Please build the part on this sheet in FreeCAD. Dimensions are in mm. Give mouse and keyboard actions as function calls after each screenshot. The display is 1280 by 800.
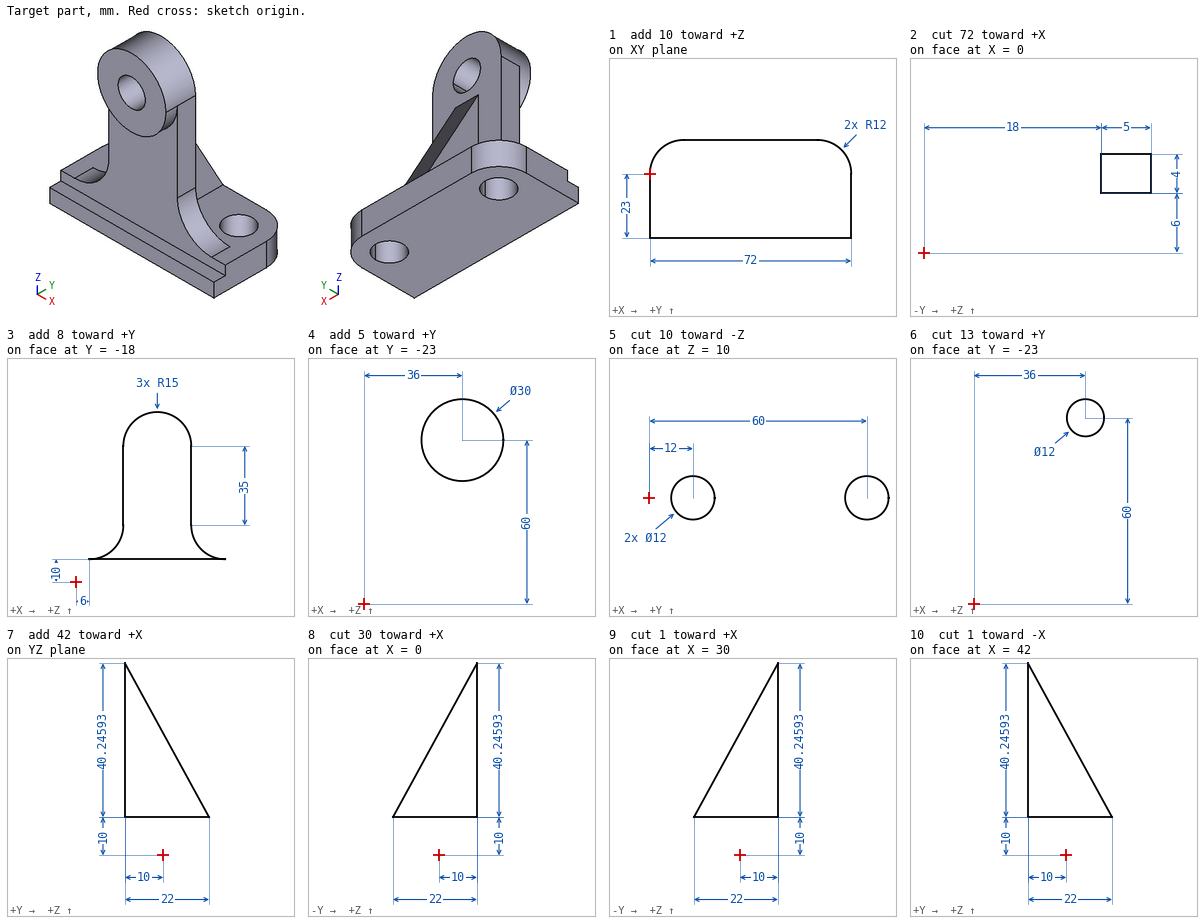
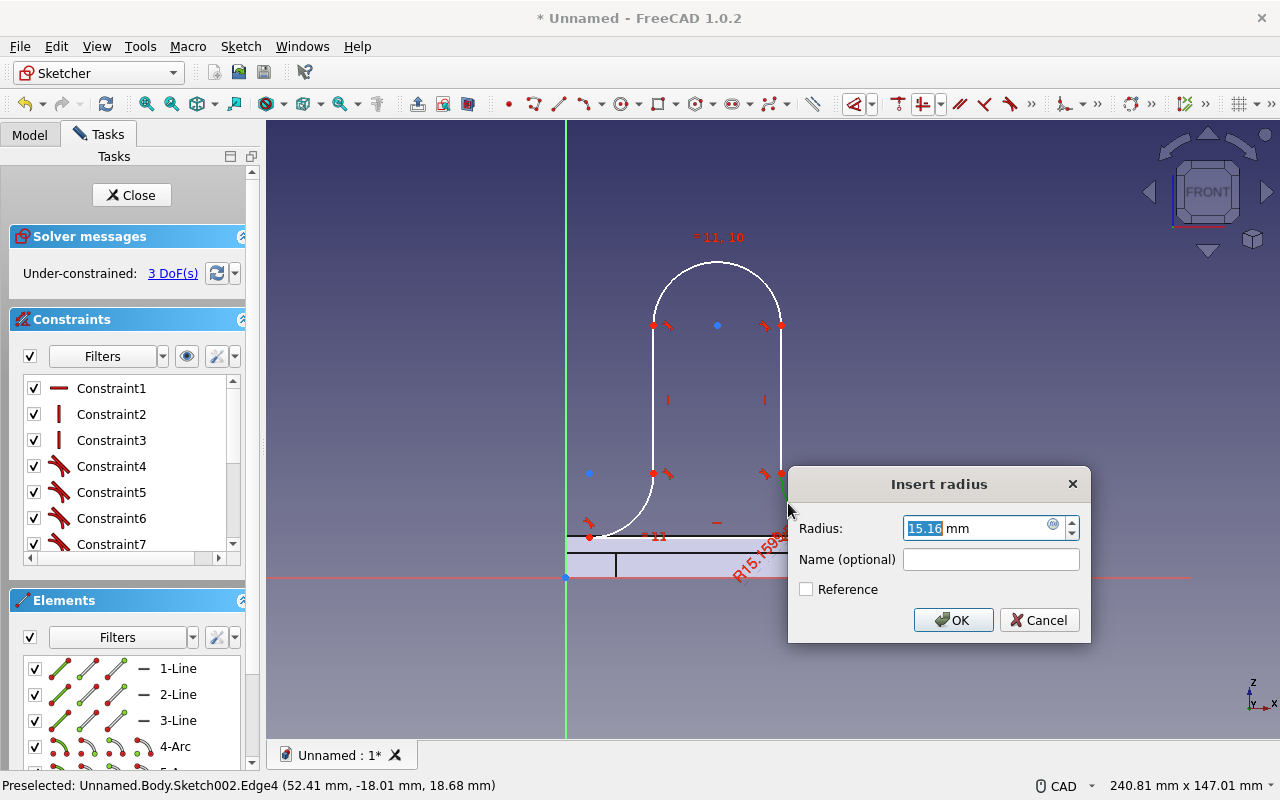
text(15)
key(Return)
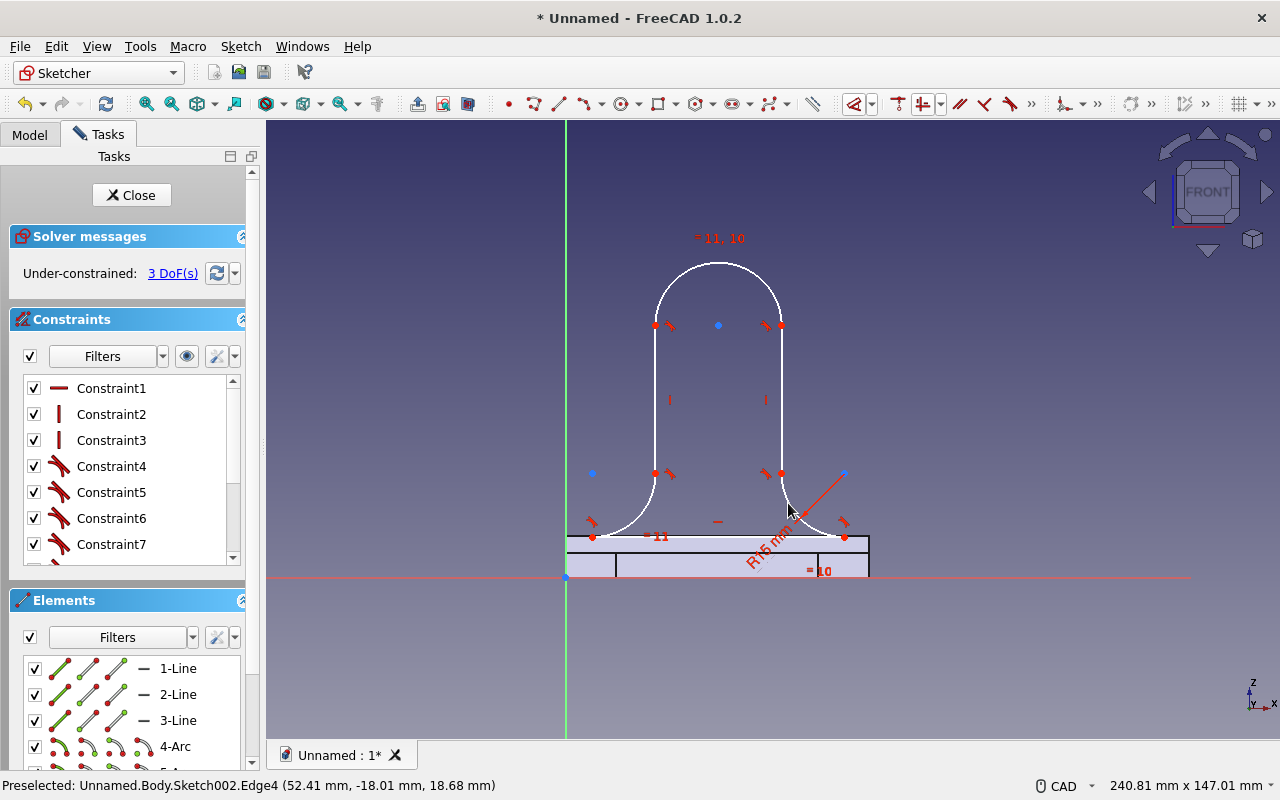
click(782, 430)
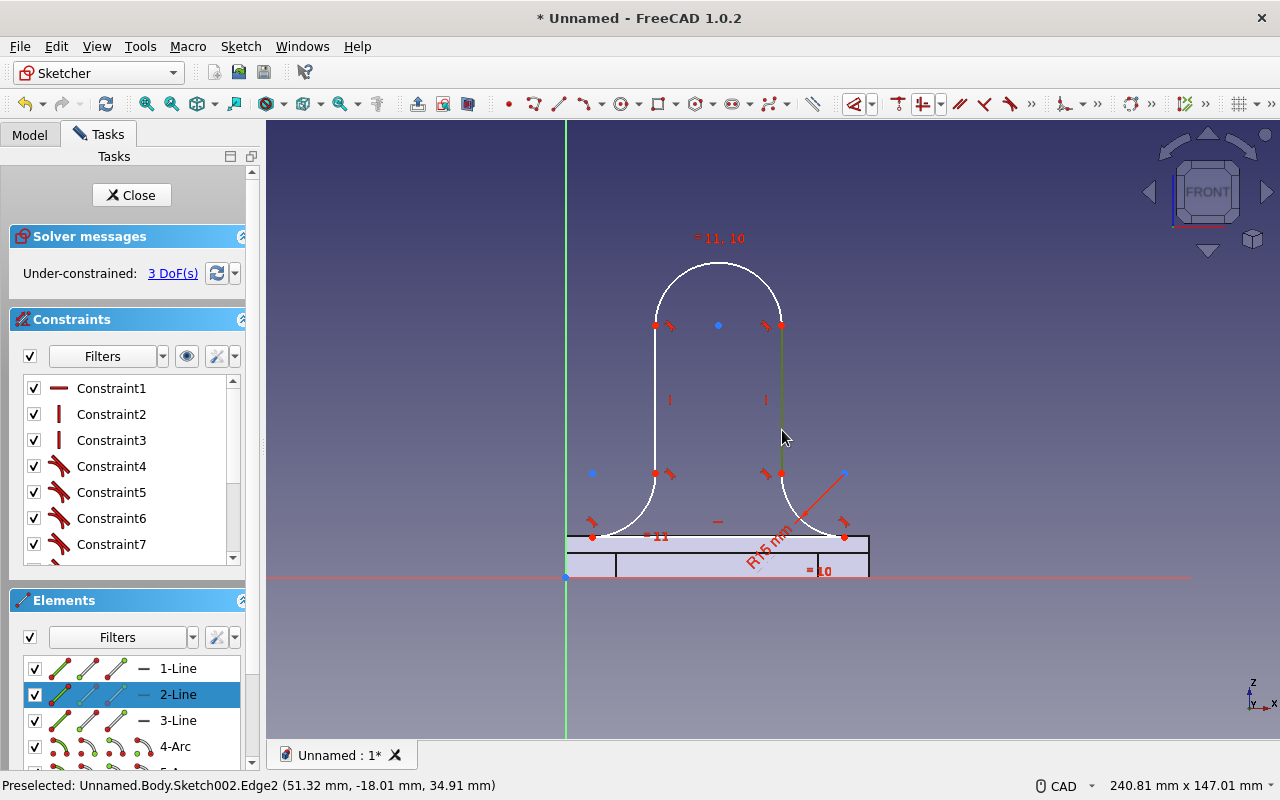
click(872, 104)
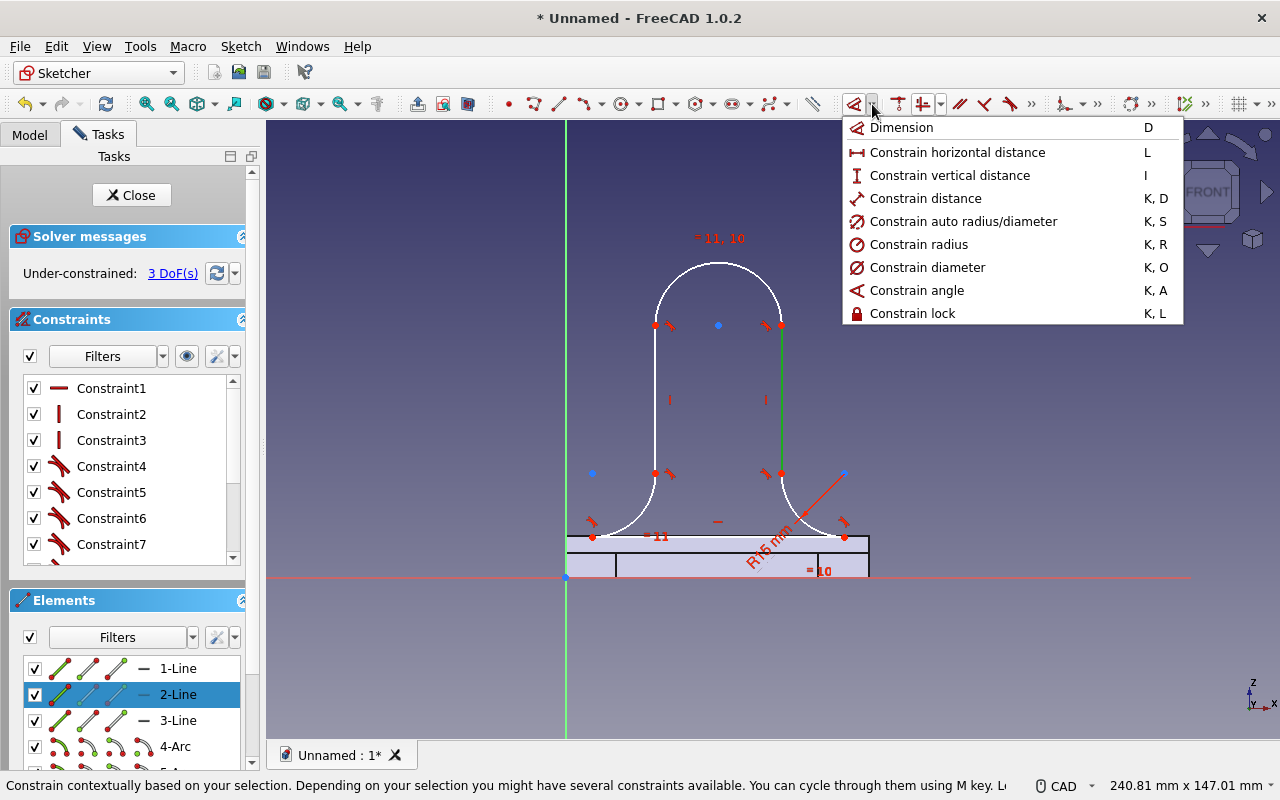
click(1013, 176)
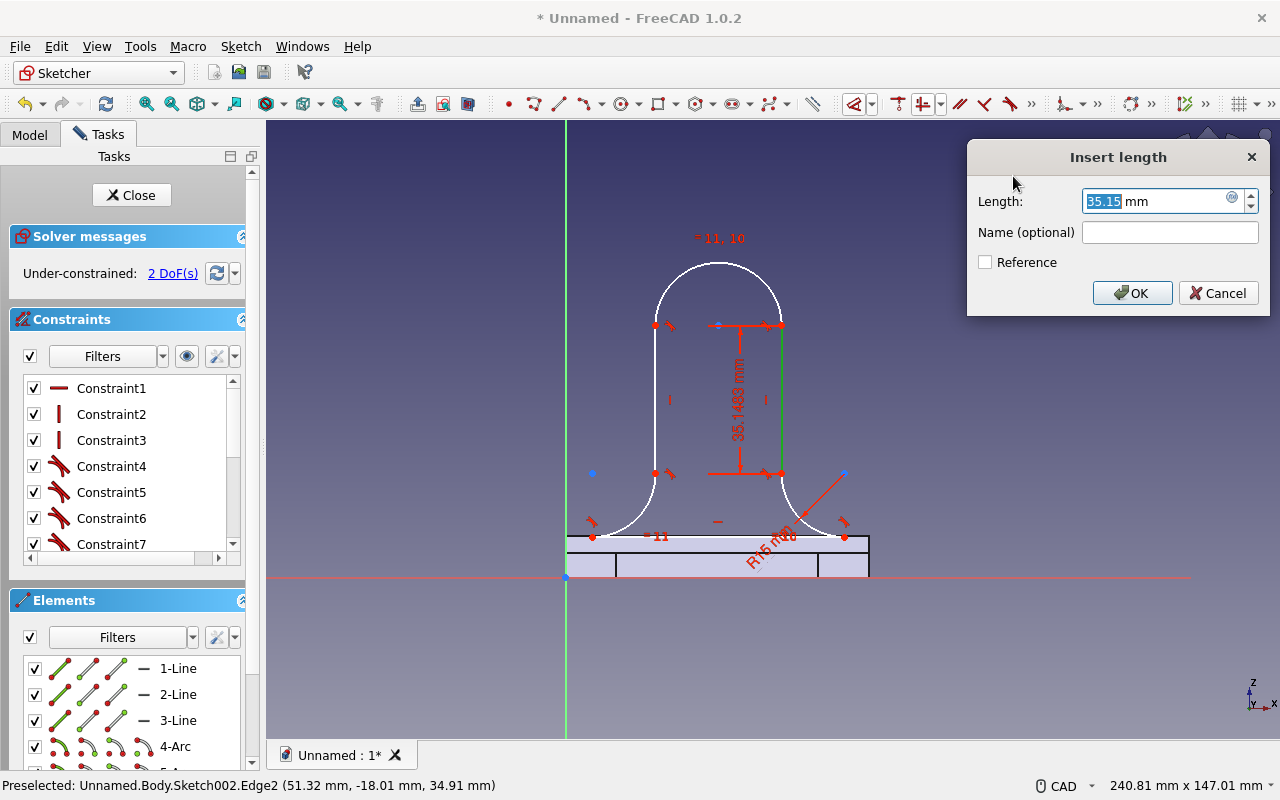
text(35)
key(Return)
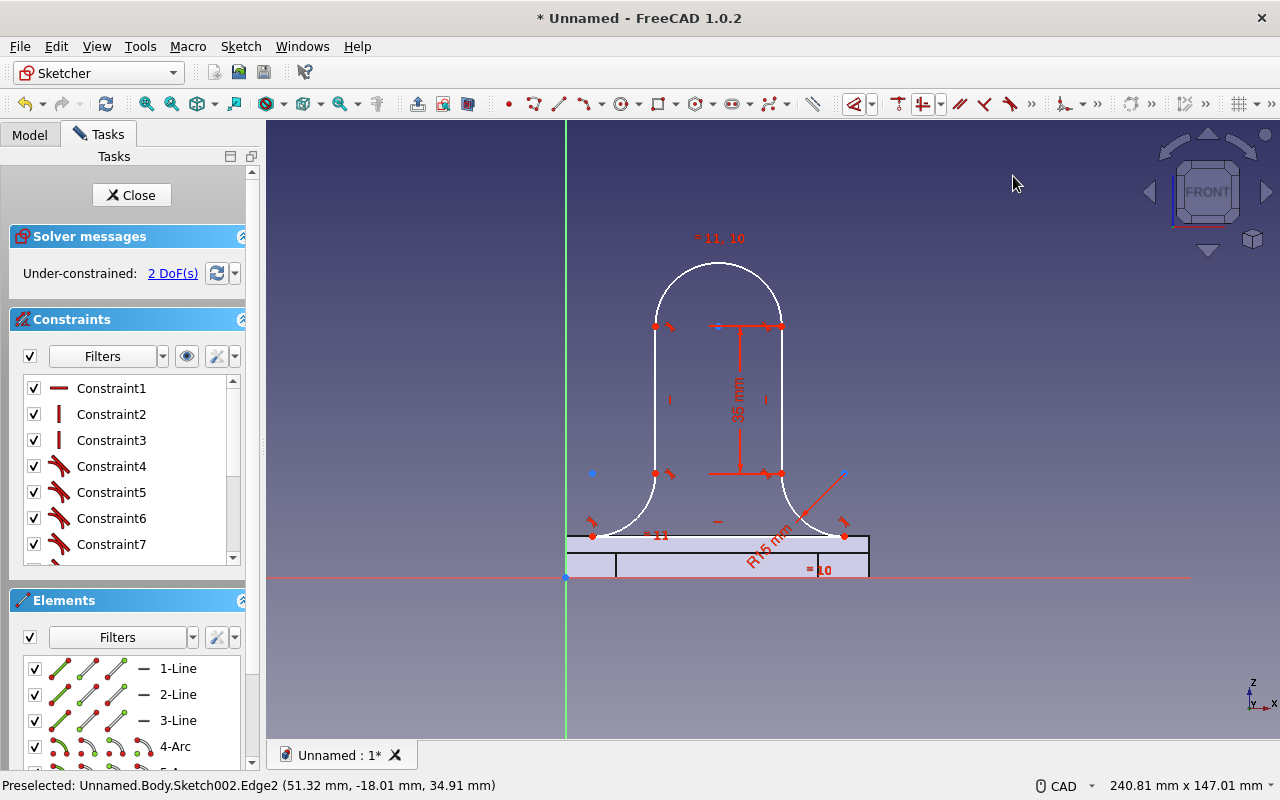
scroll(592, 537, up, 3)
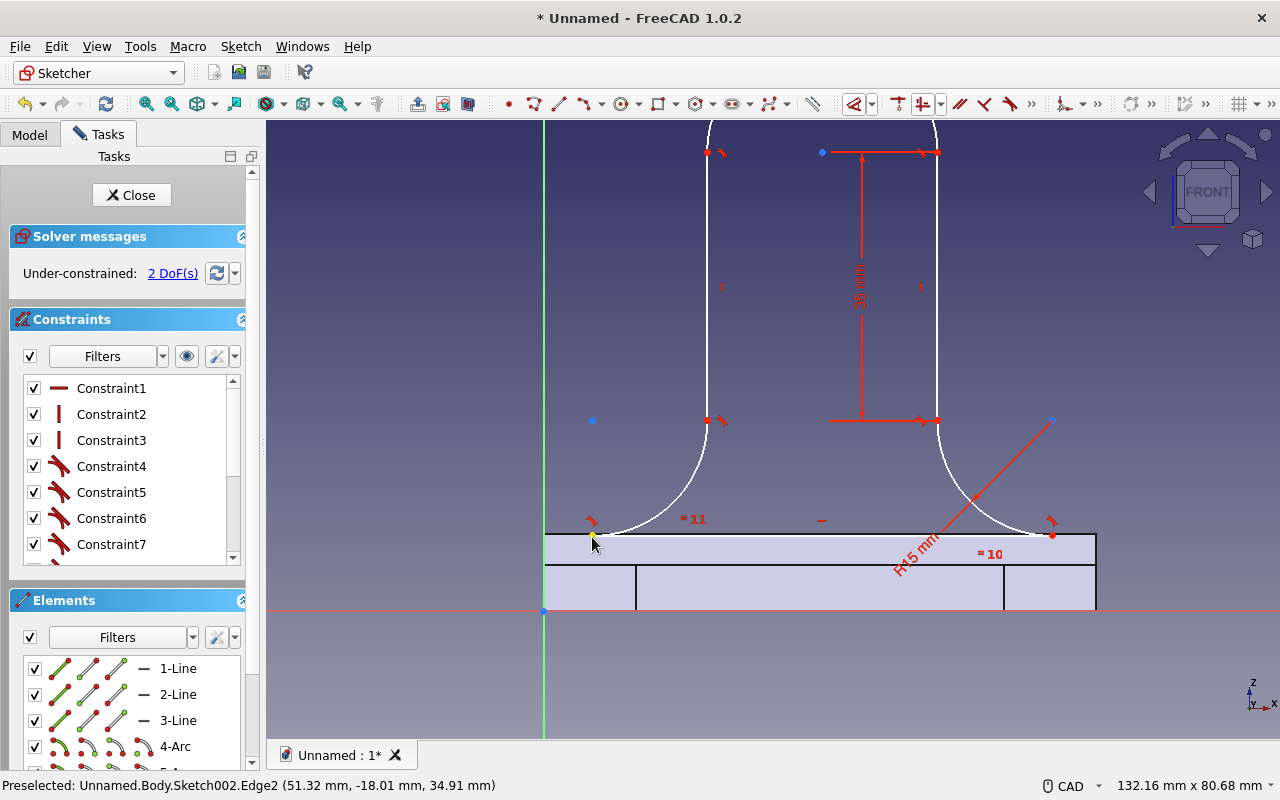
click(592, 536)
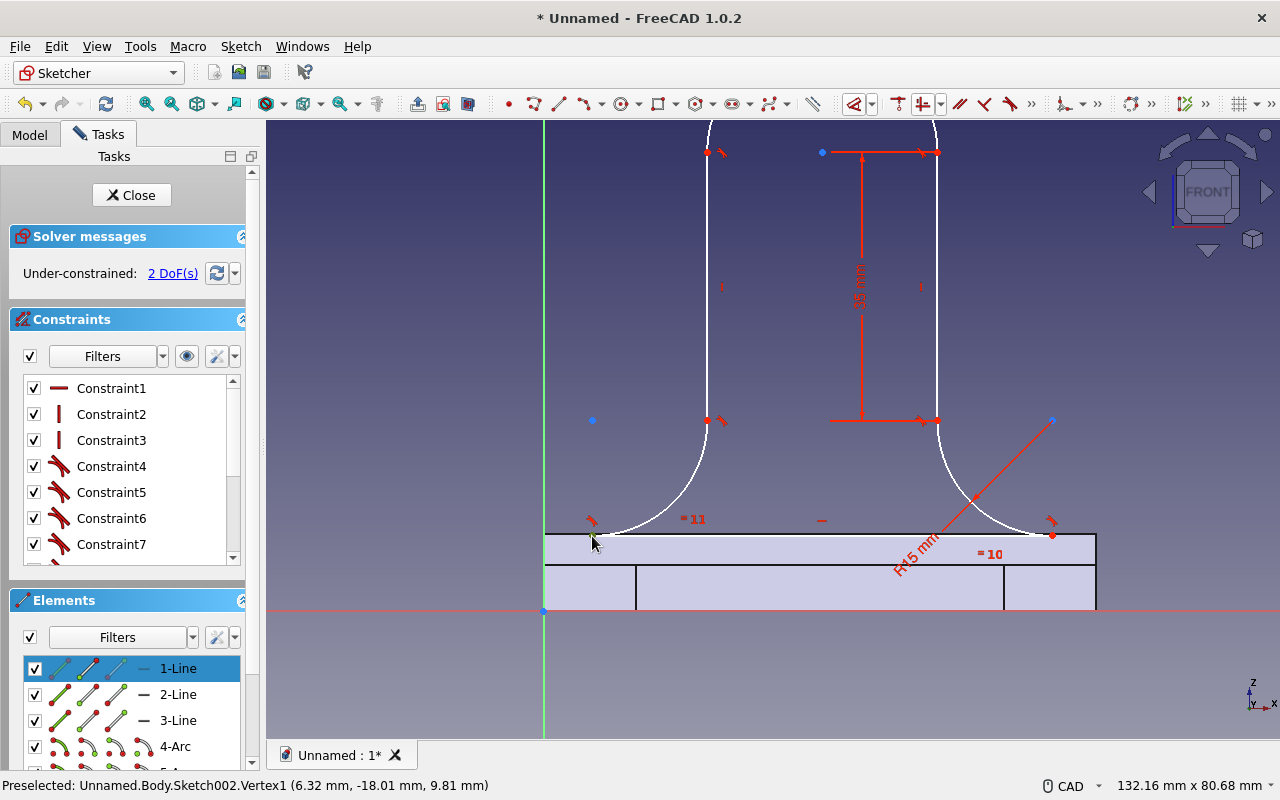
key(l)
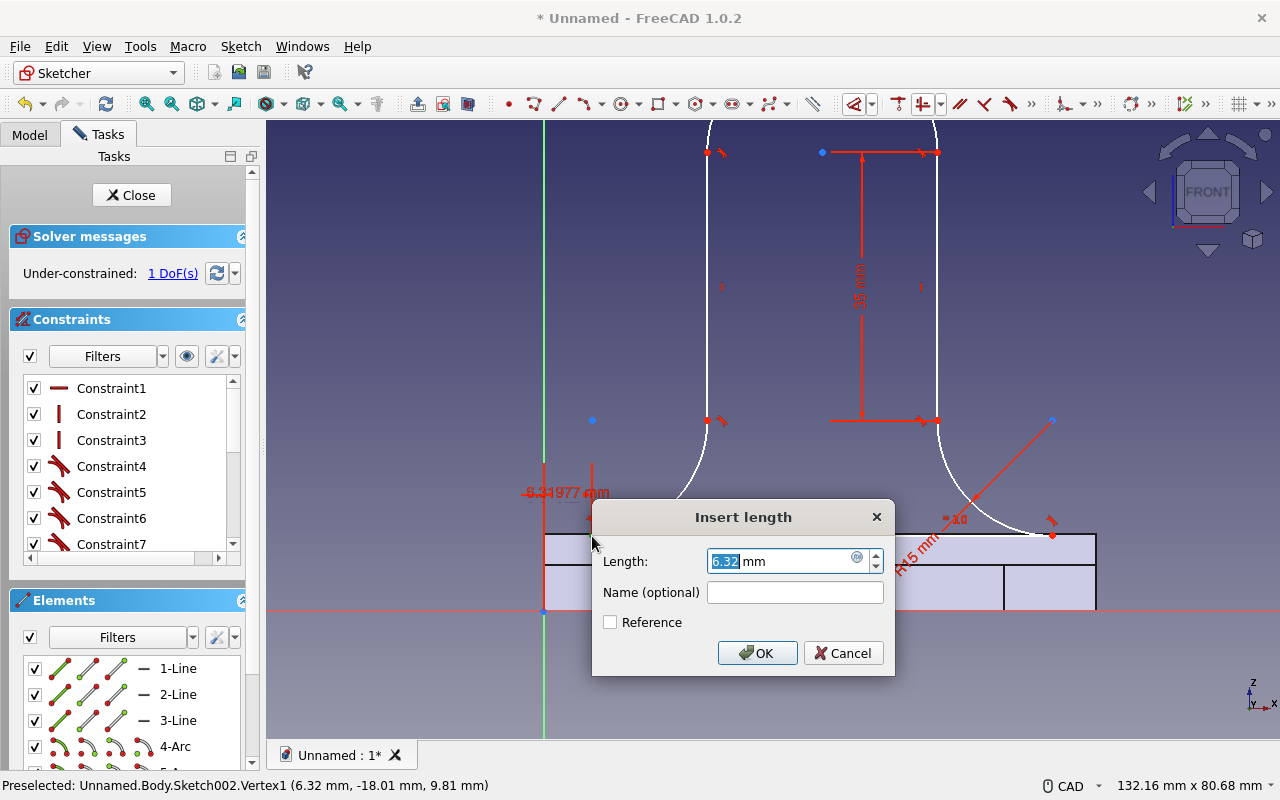
text(6)
key(Return)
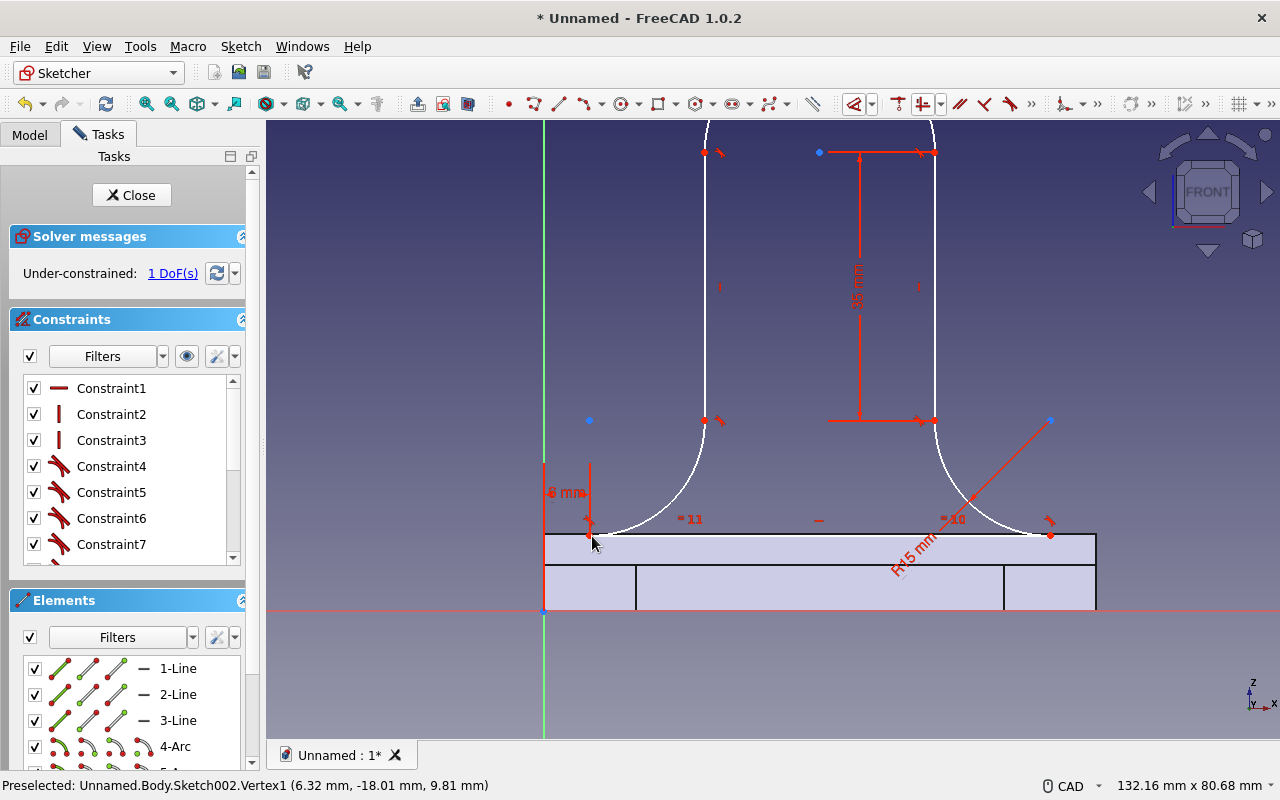
click(590, 536)